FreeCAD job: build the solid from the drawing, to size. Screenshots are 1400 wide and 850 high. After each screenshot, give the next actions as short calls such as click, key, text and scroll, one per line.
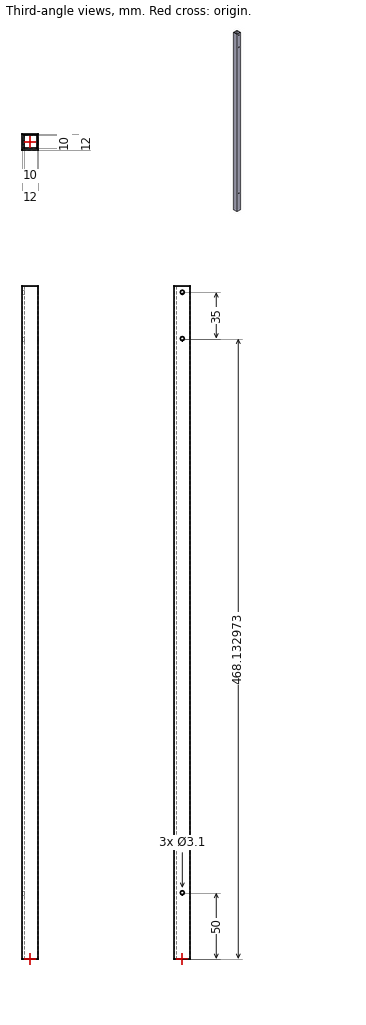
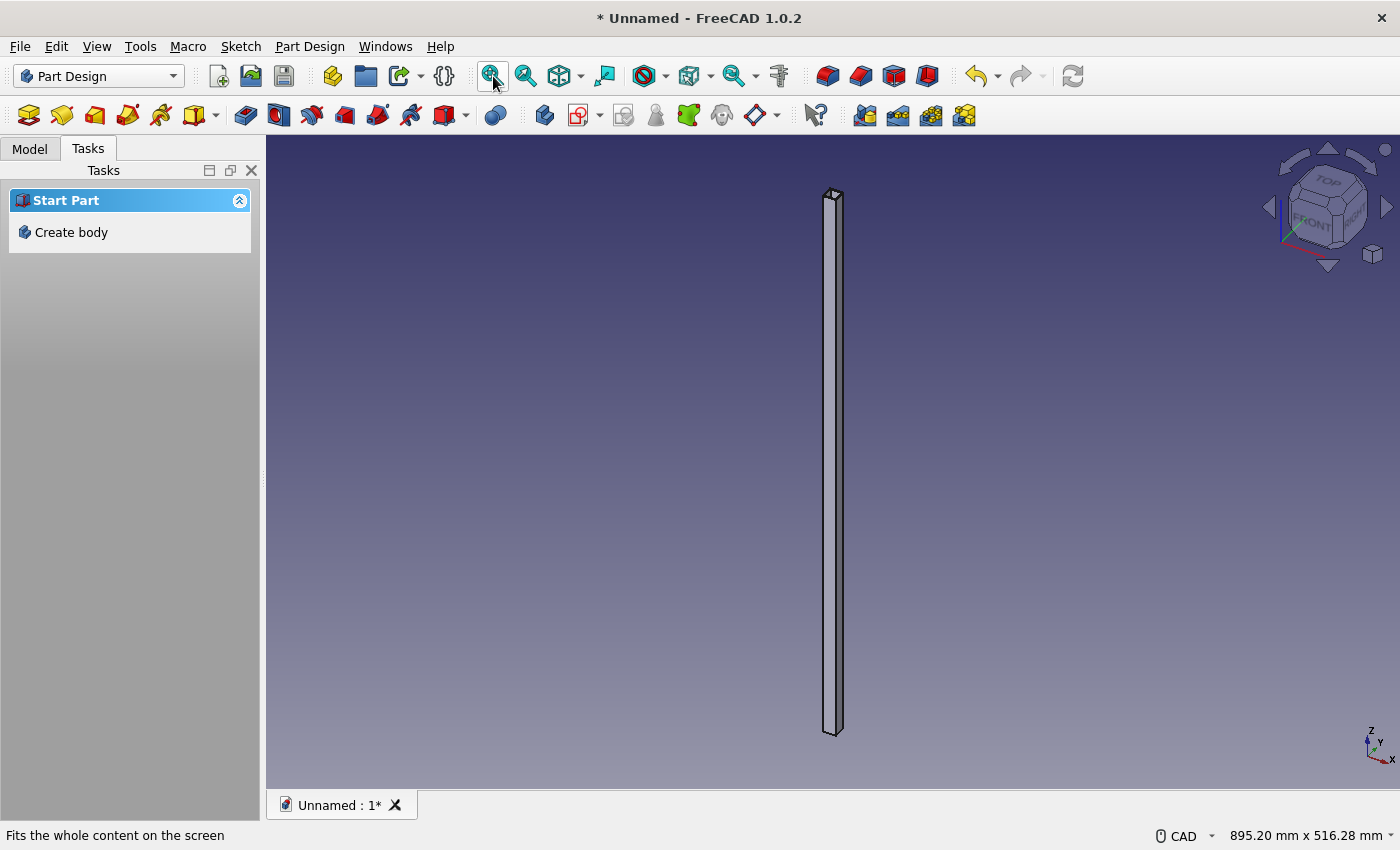
key(6)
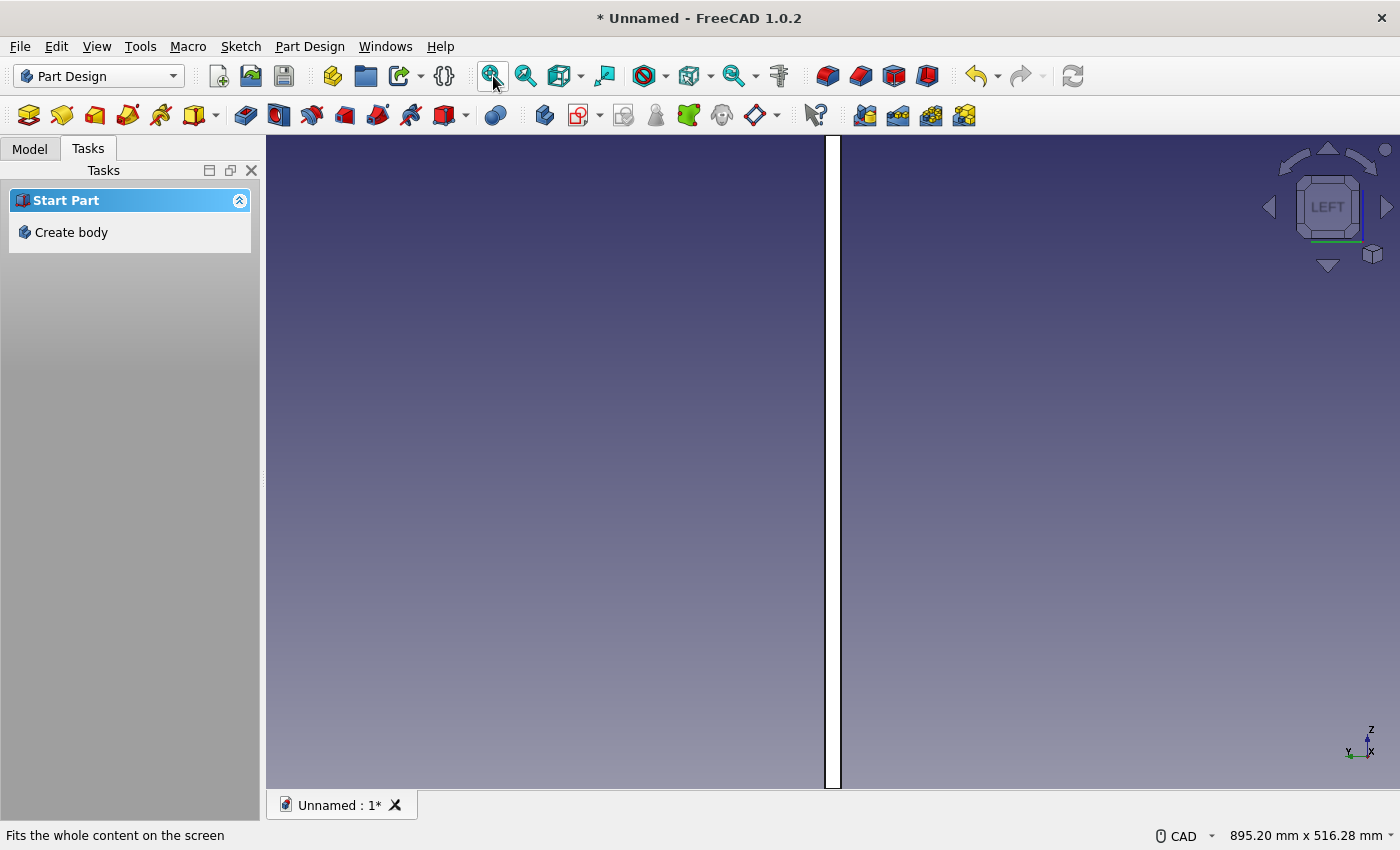
click(493, 76)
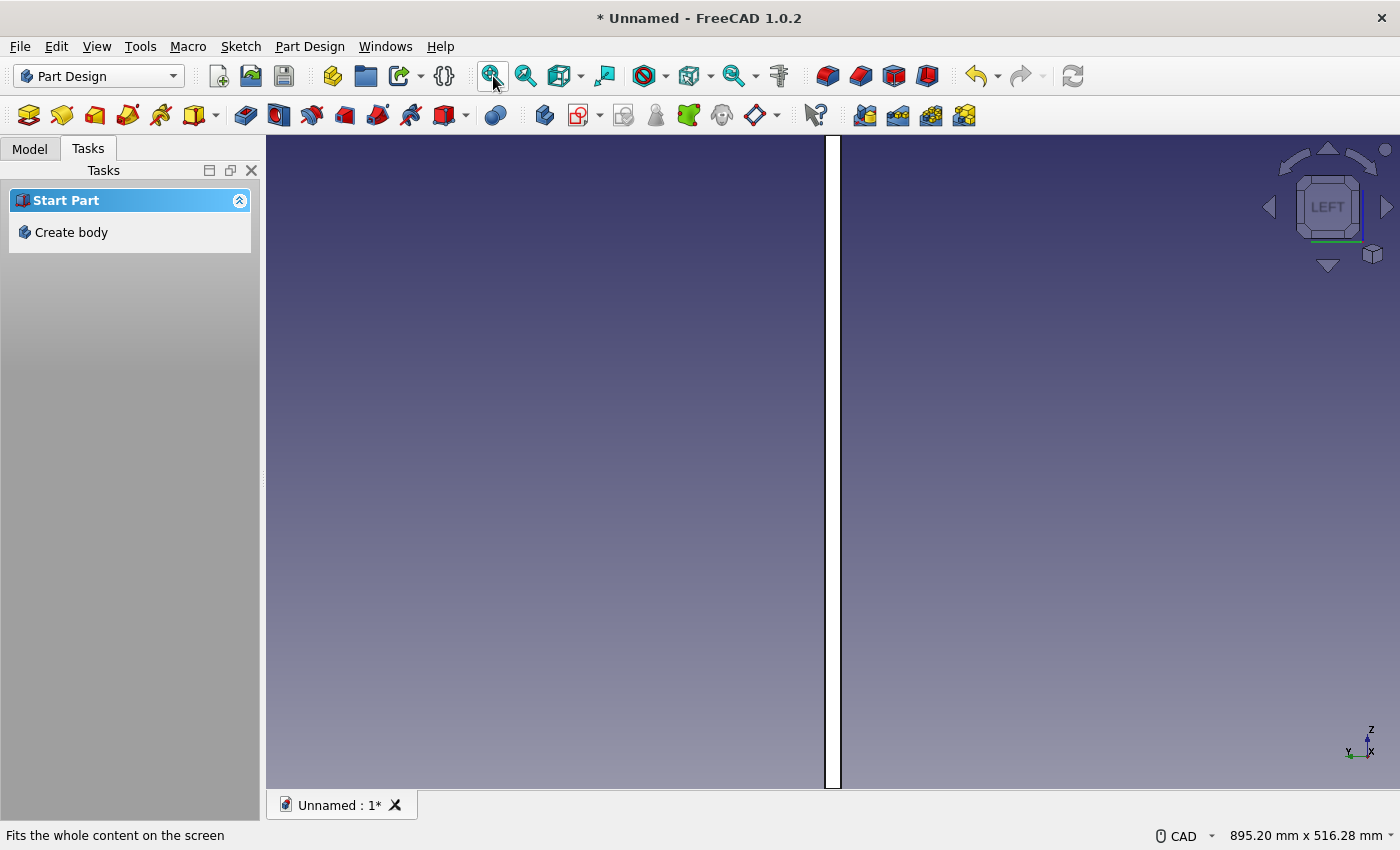
key(2)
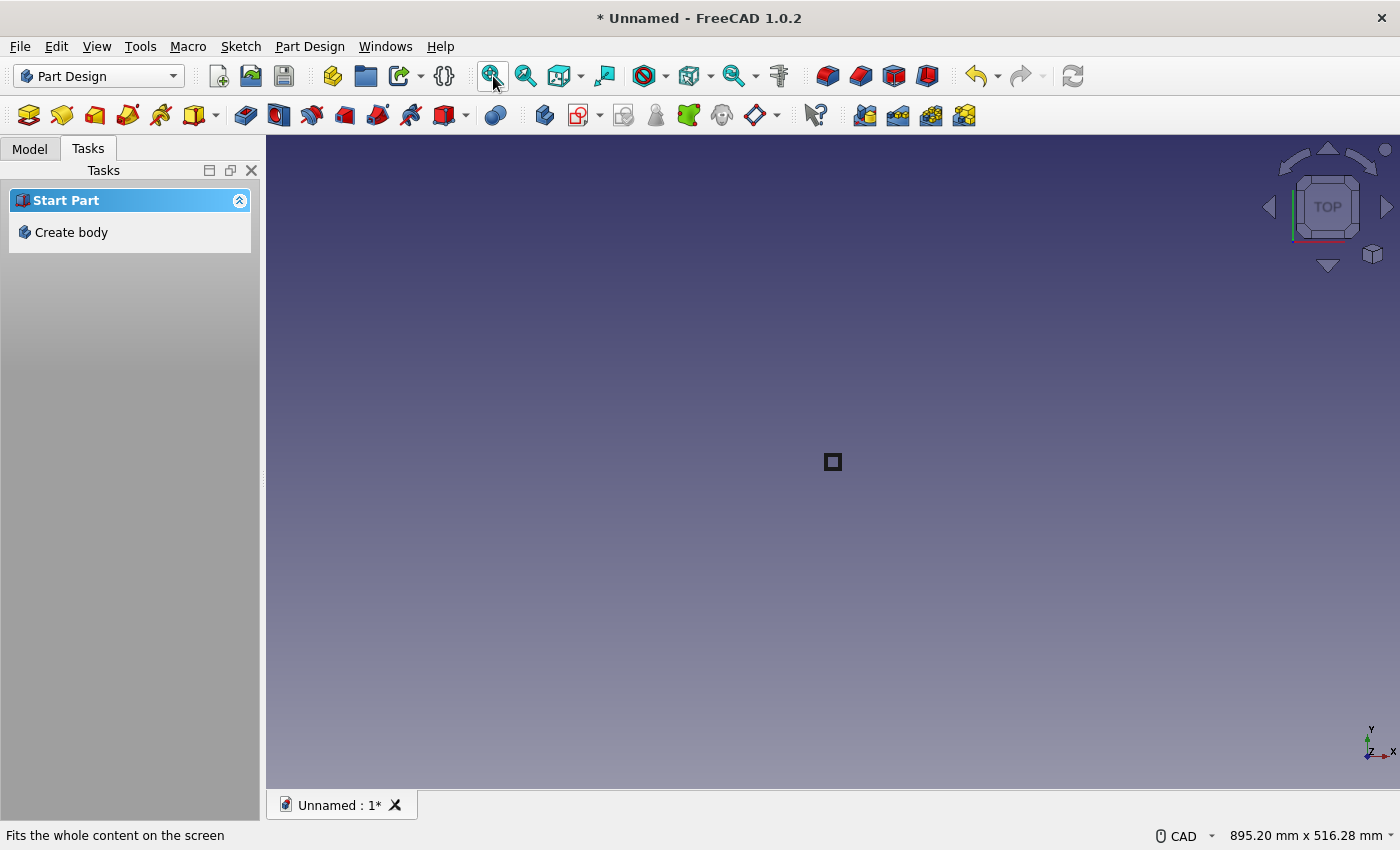
click(493, 76)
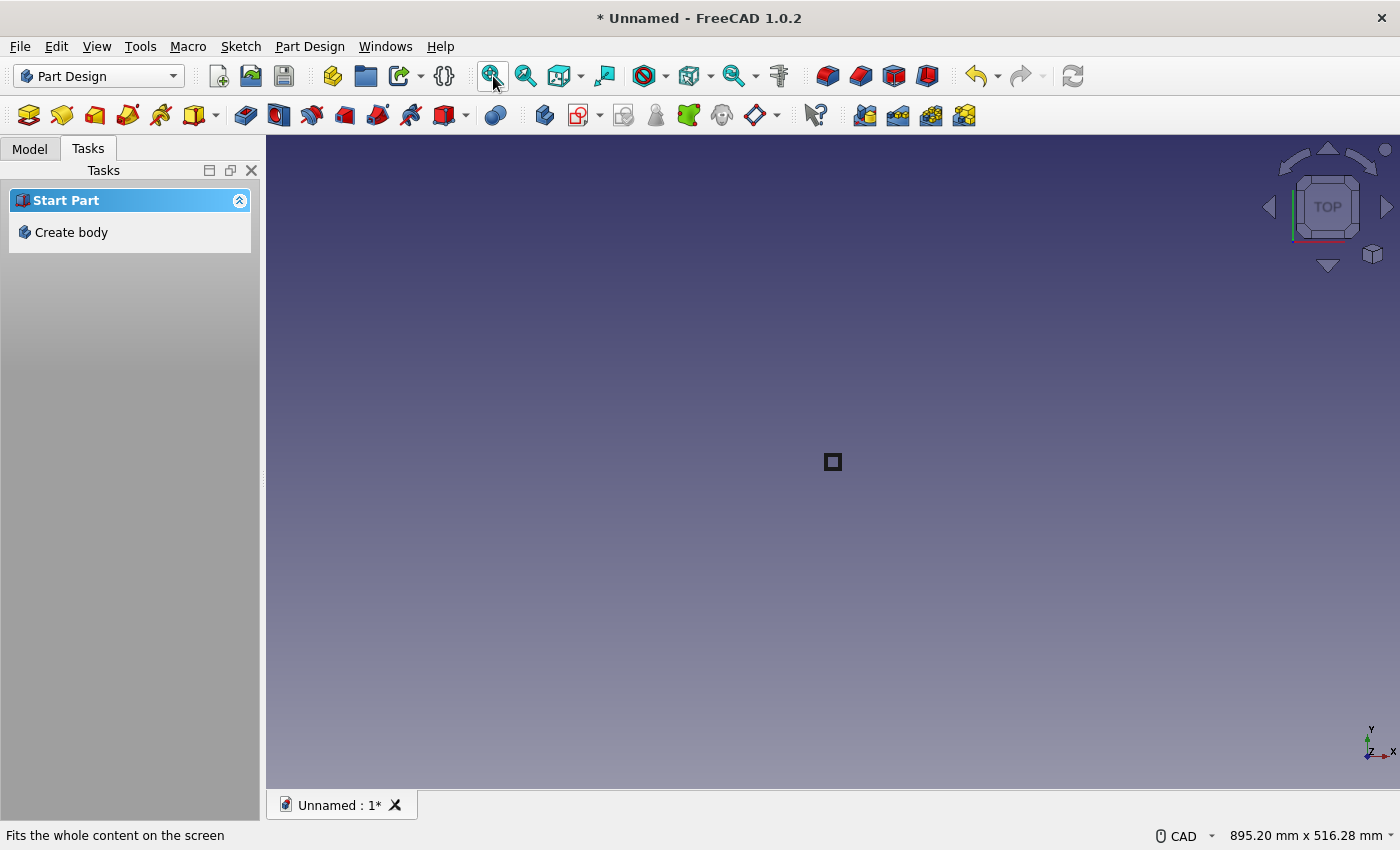
key(1)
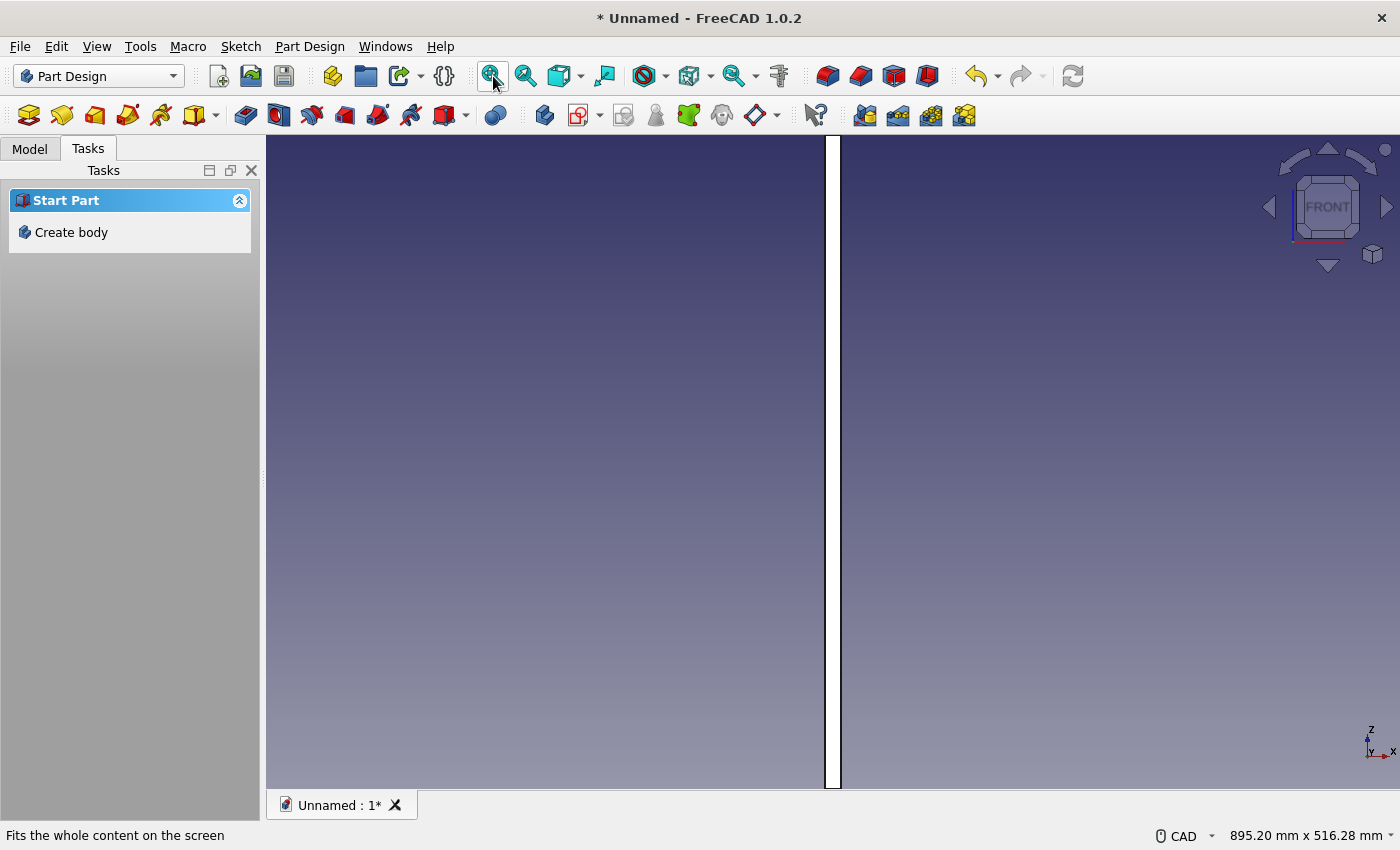
click(493, 76)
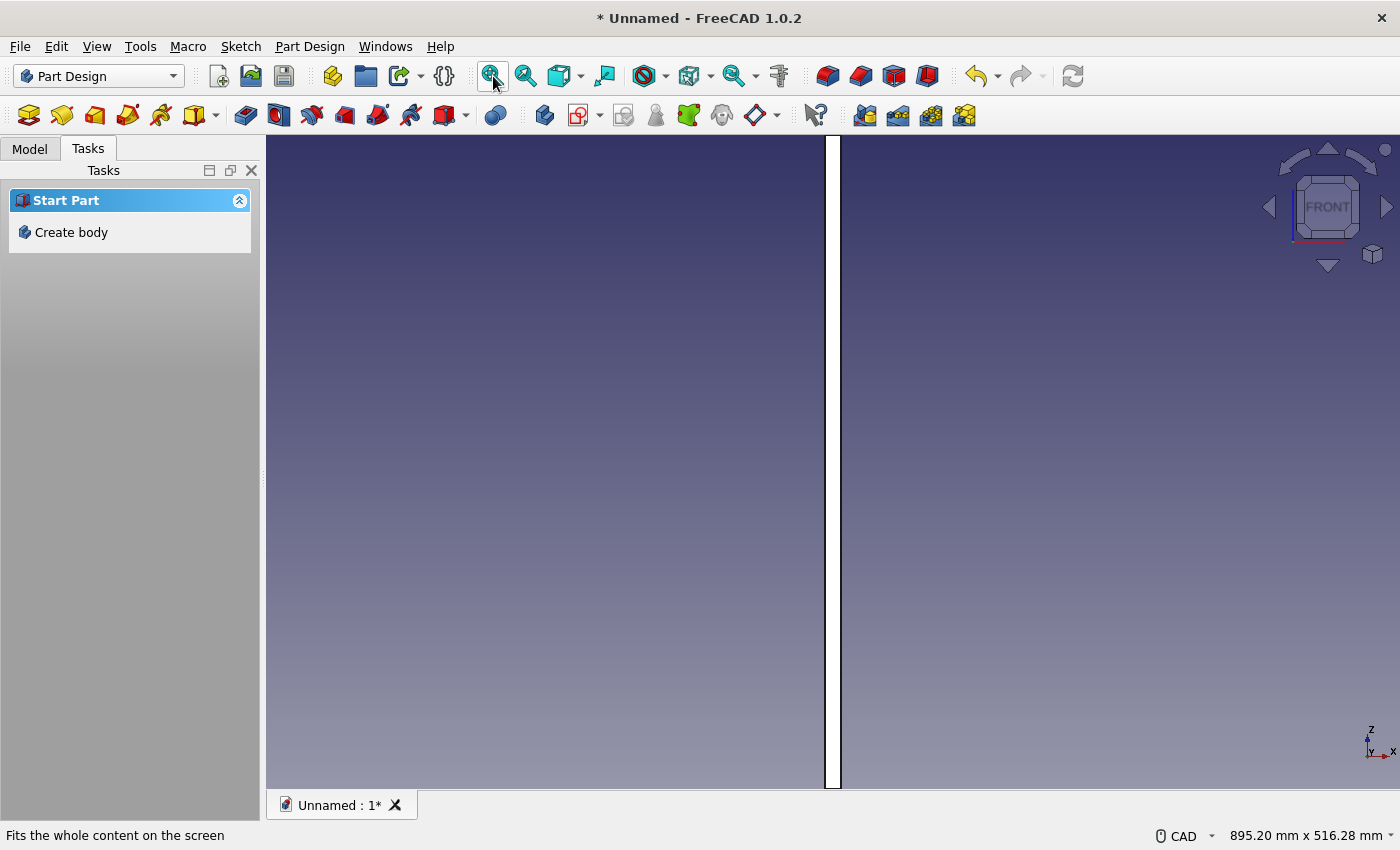
click(30, 148)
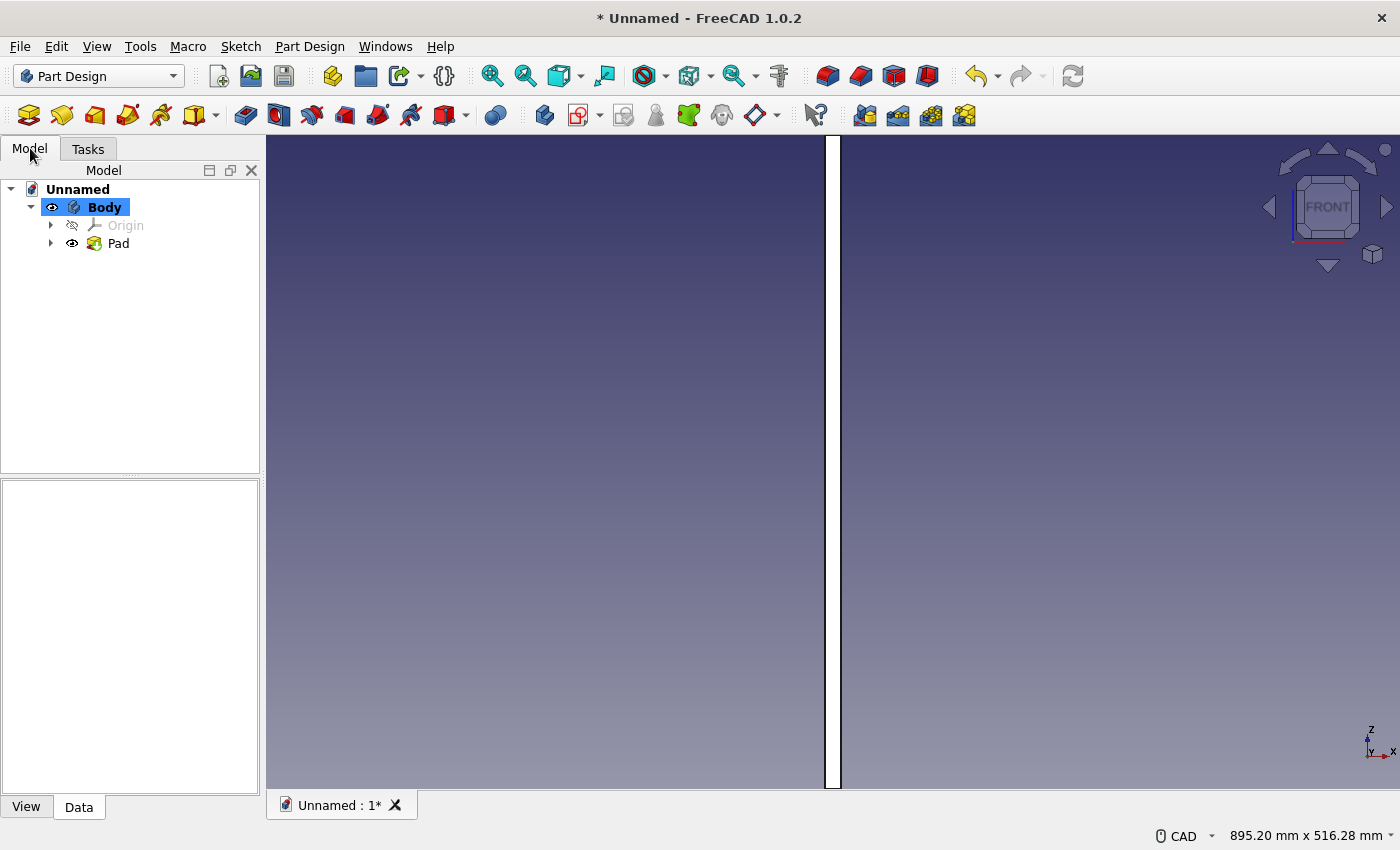
click(51, 225)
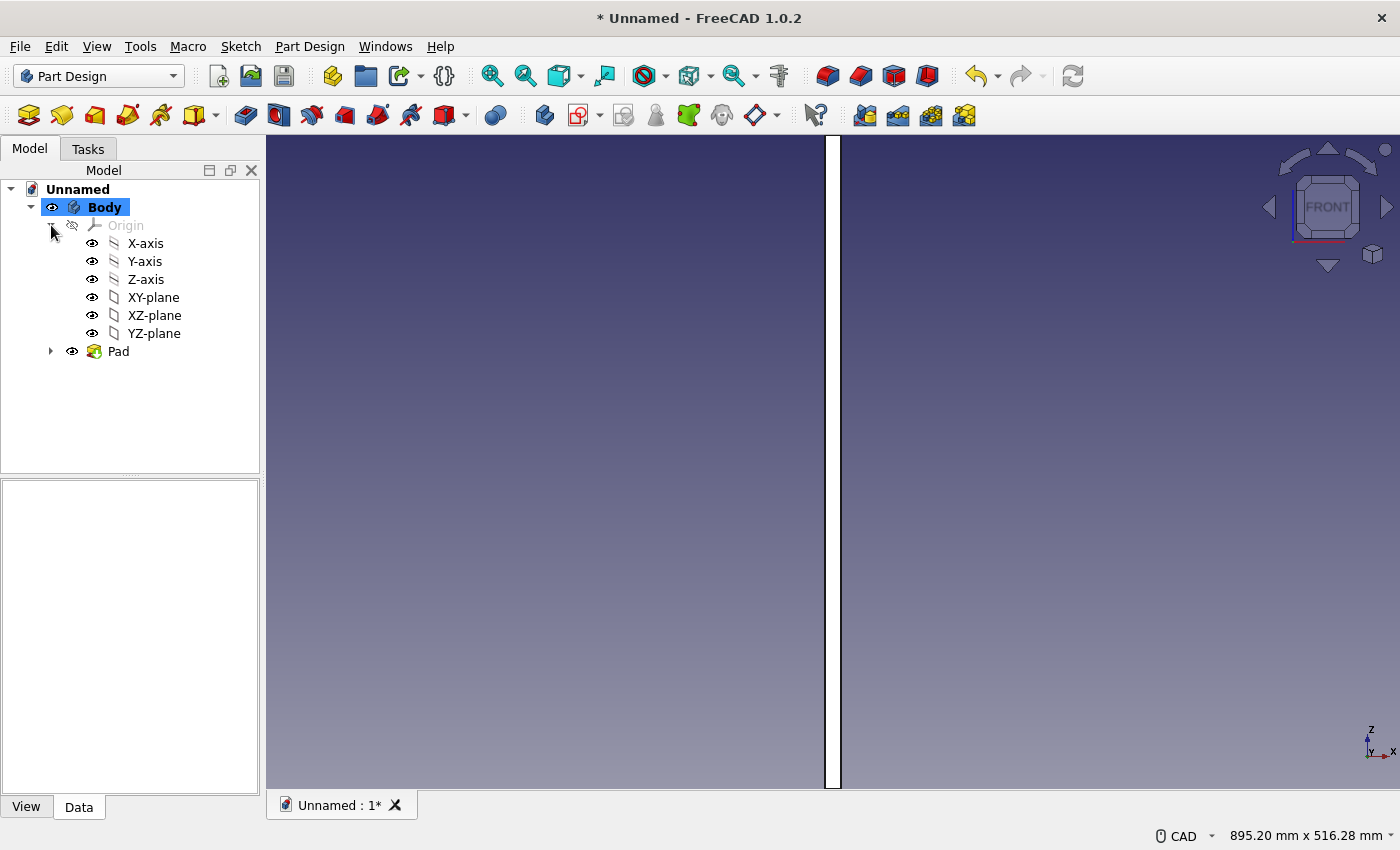
click(137, 333)